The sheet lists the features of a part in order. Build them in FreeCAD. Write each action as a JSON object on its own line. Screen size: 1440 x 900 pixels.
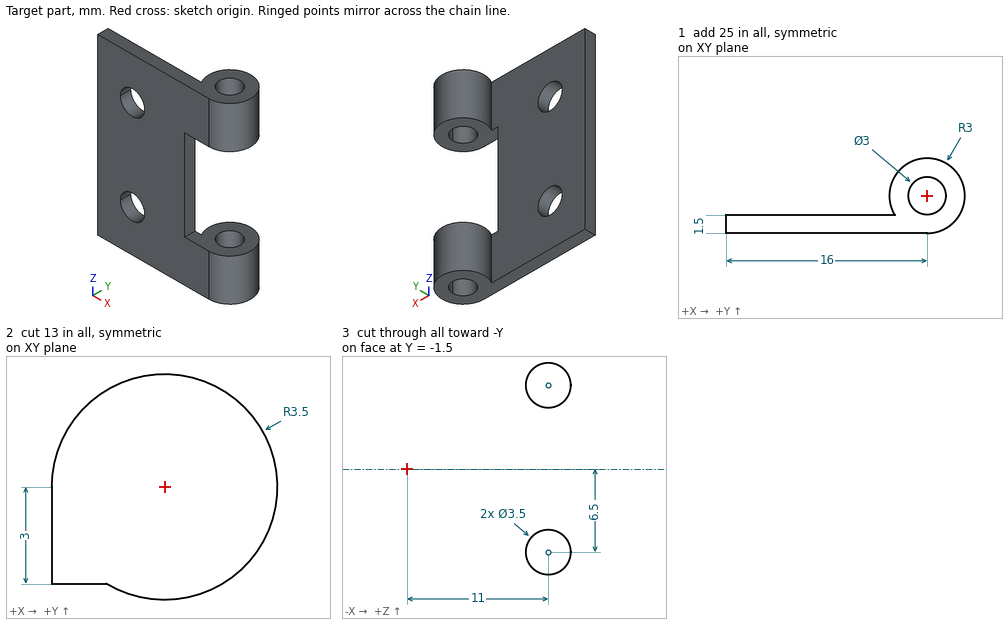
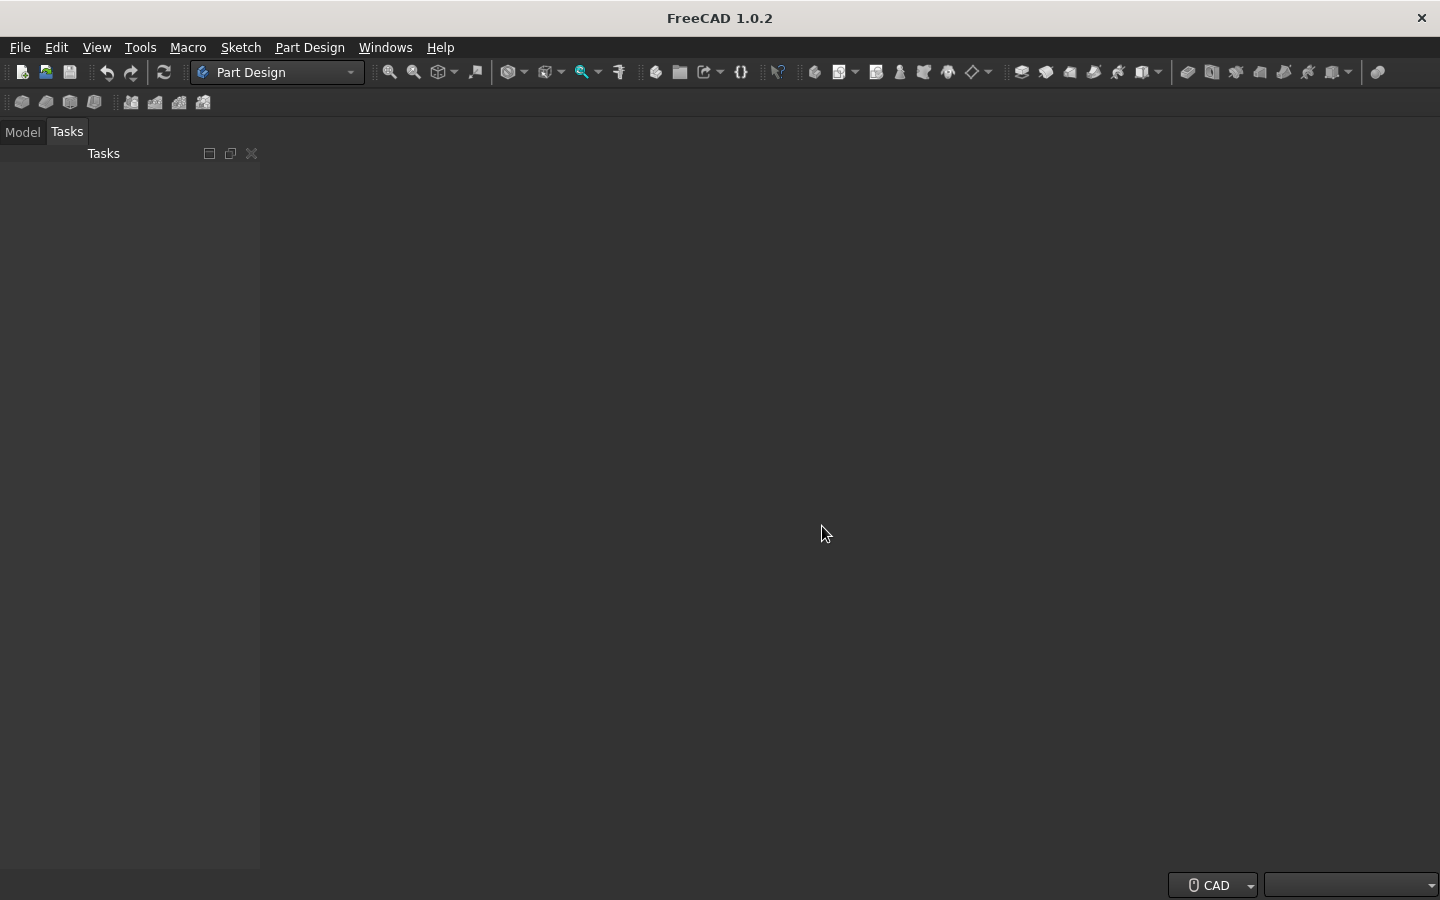
{"action": "left_click", "coordinate": [22, 72]}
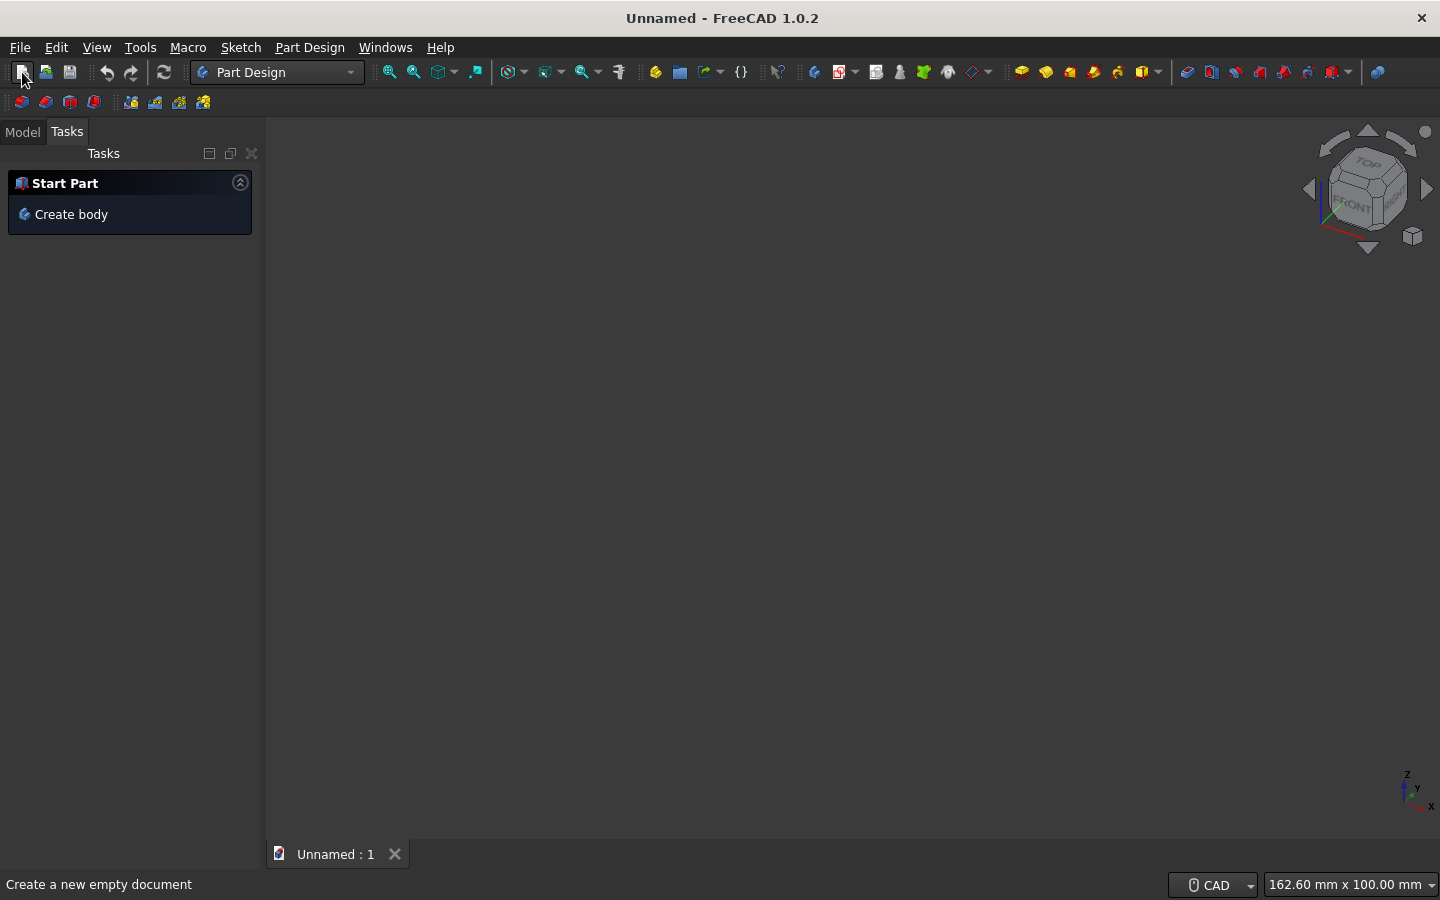
{"action": "left_click", "coordinate": [840, 72]}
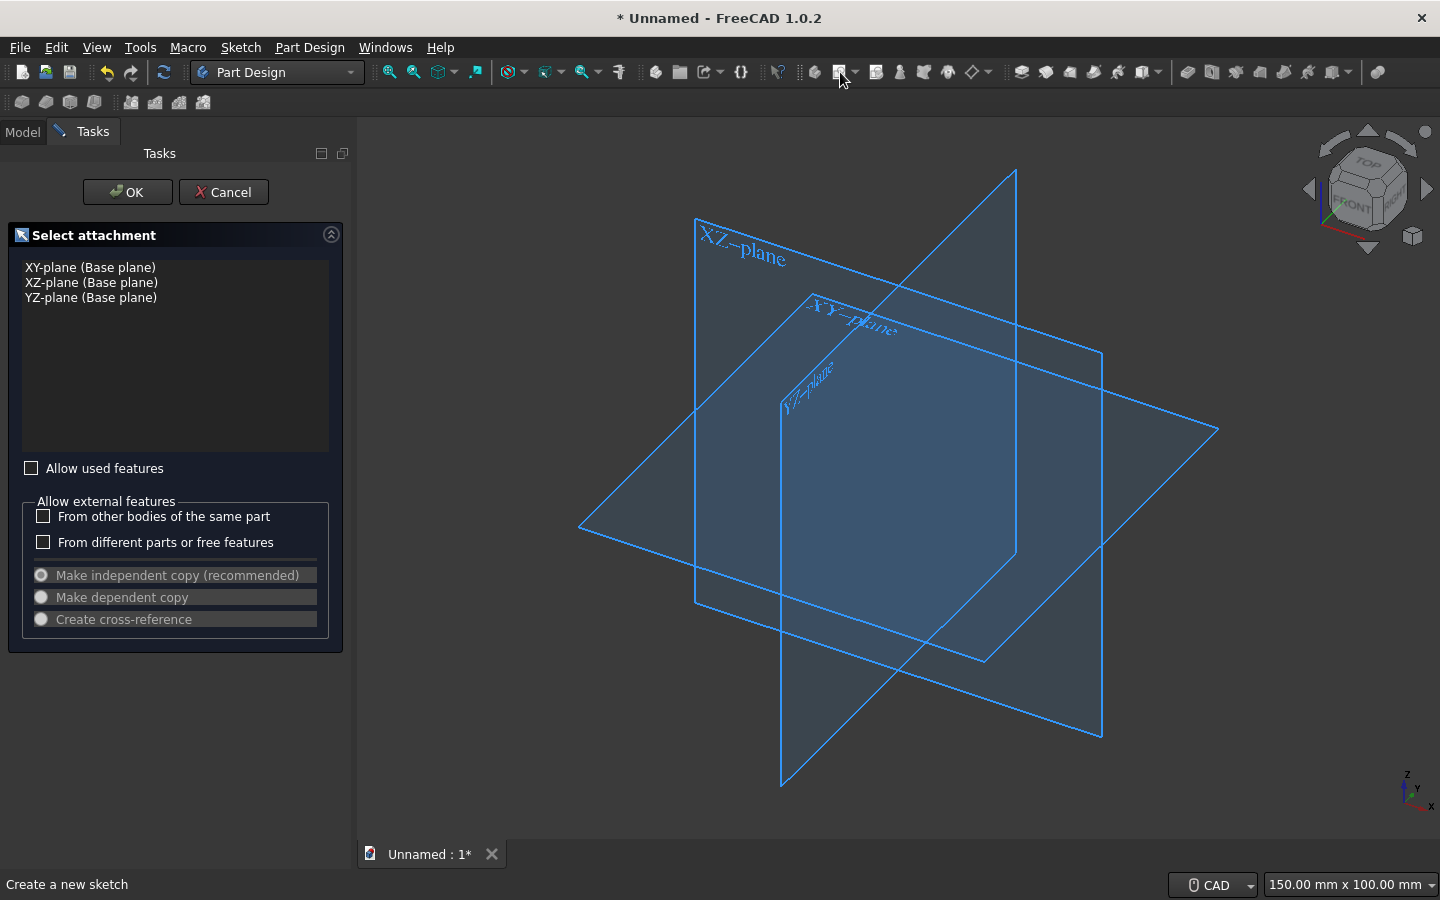
{"action": "left_click", "coordinate": [82, 268]}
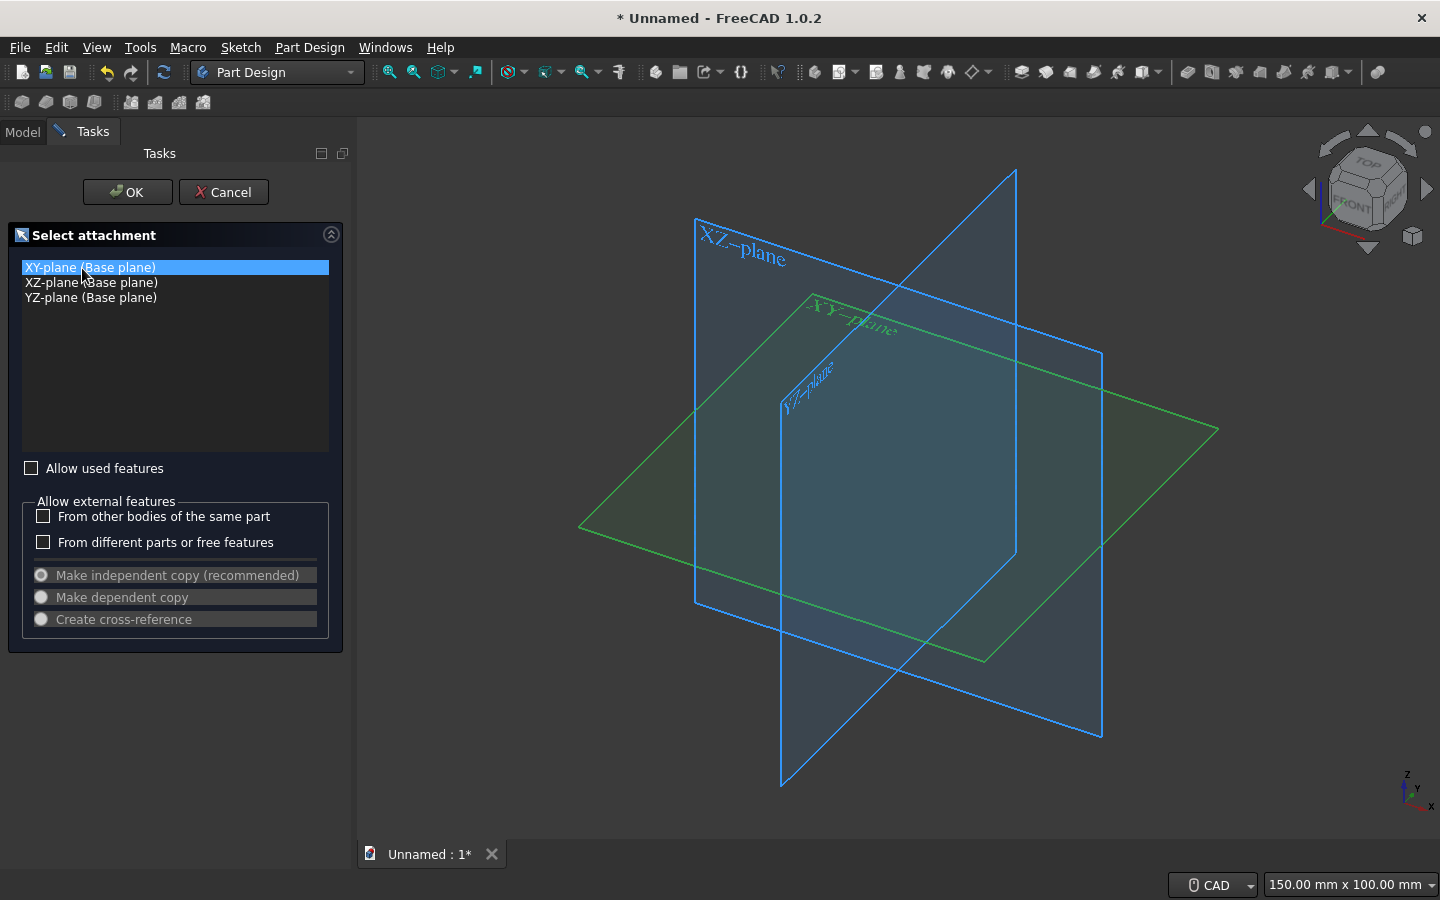
{"action": "left_click", "coordinate": [128, 192]}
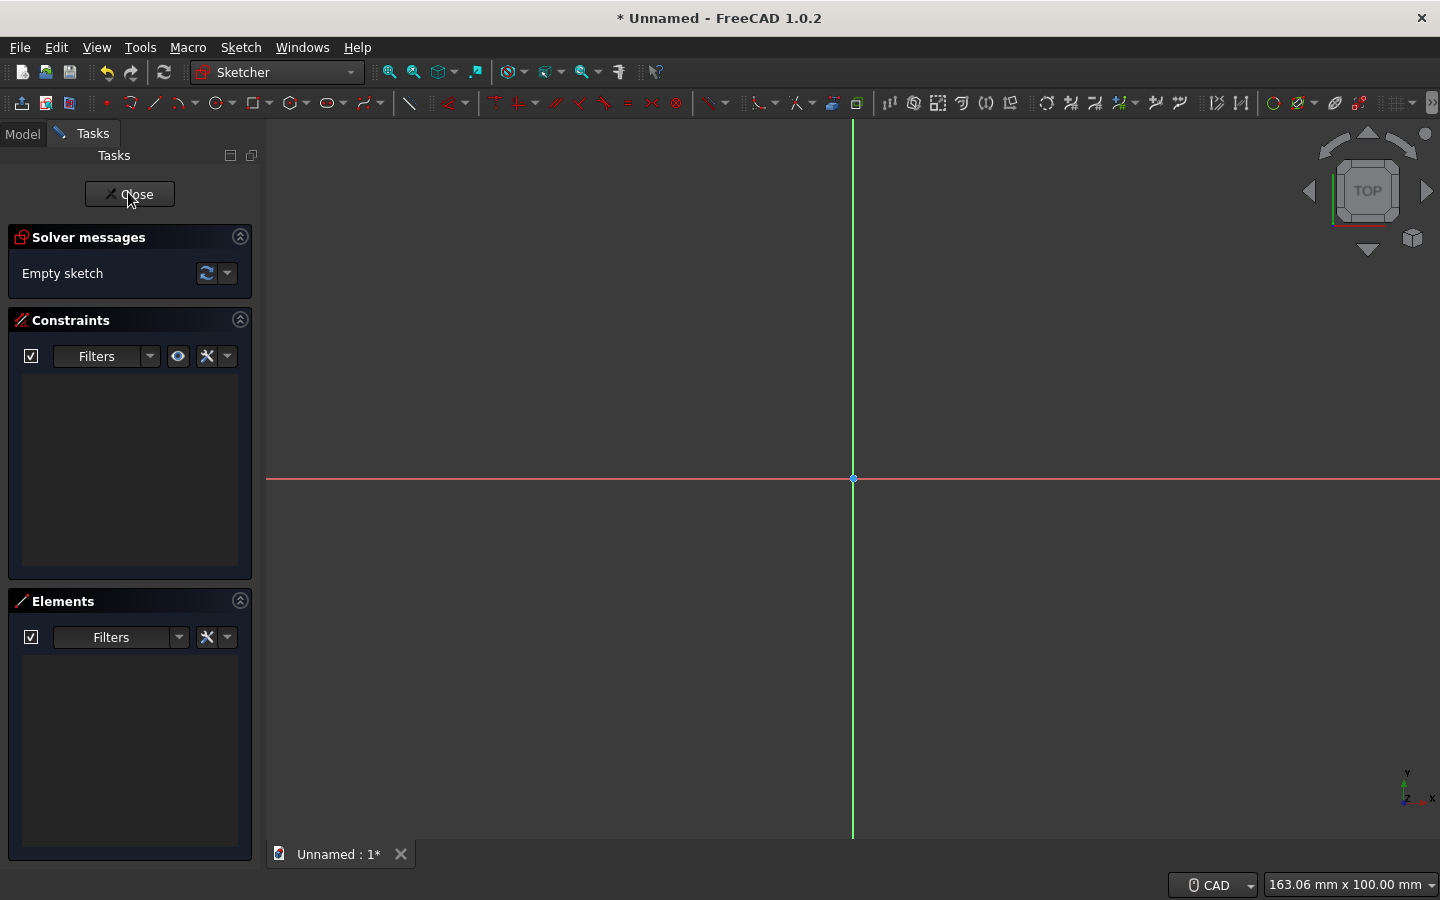
{"action": "scroll", "coordinate": [804, 481], "scroll_direction": "up", "scroll_amount": 9}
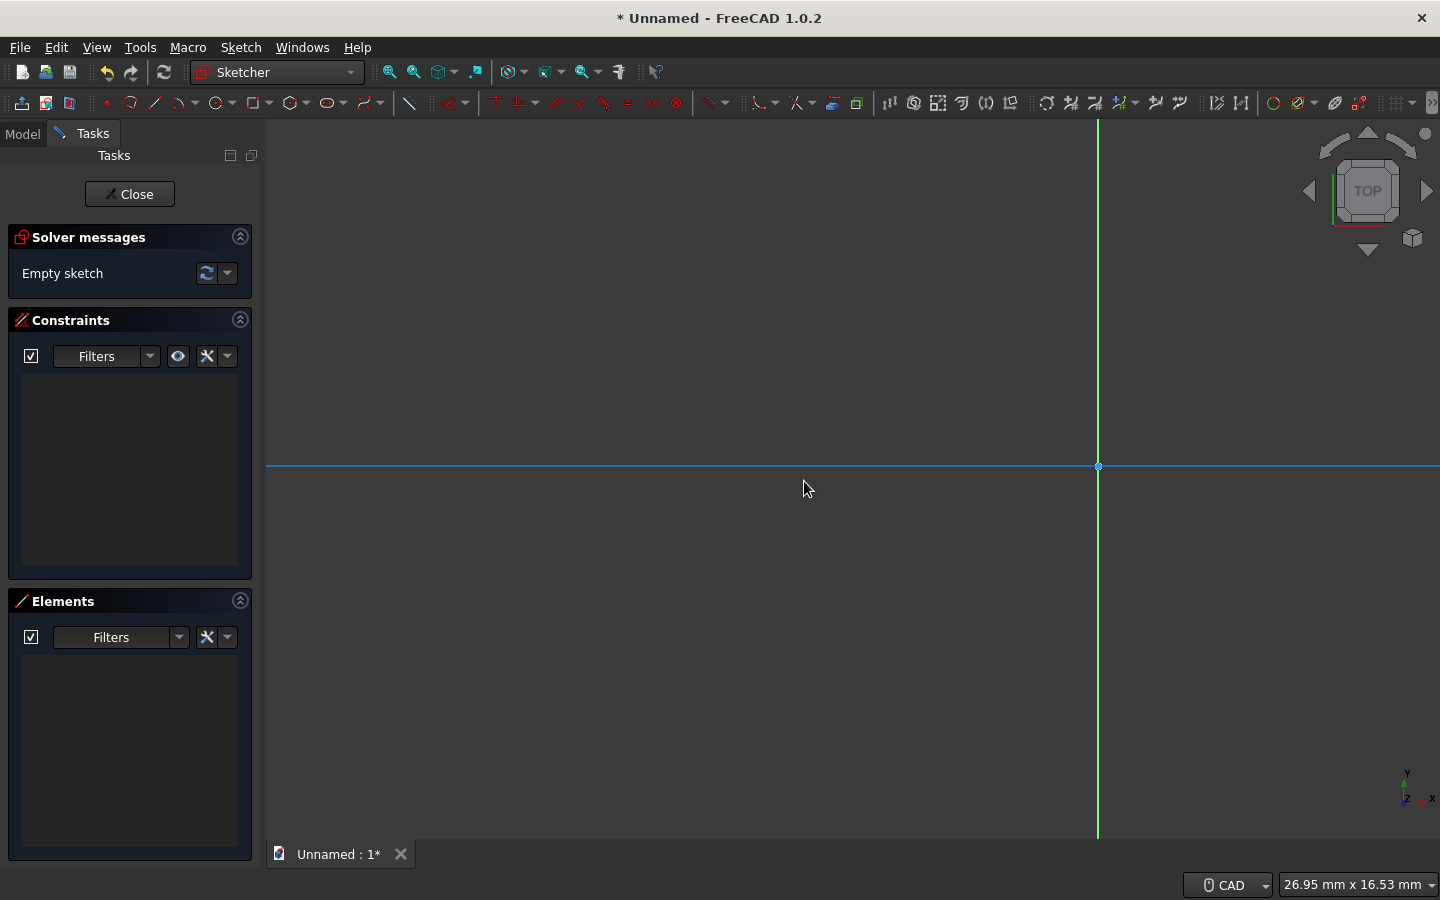
{"action": "left_click", "coordinate": [132, 104]}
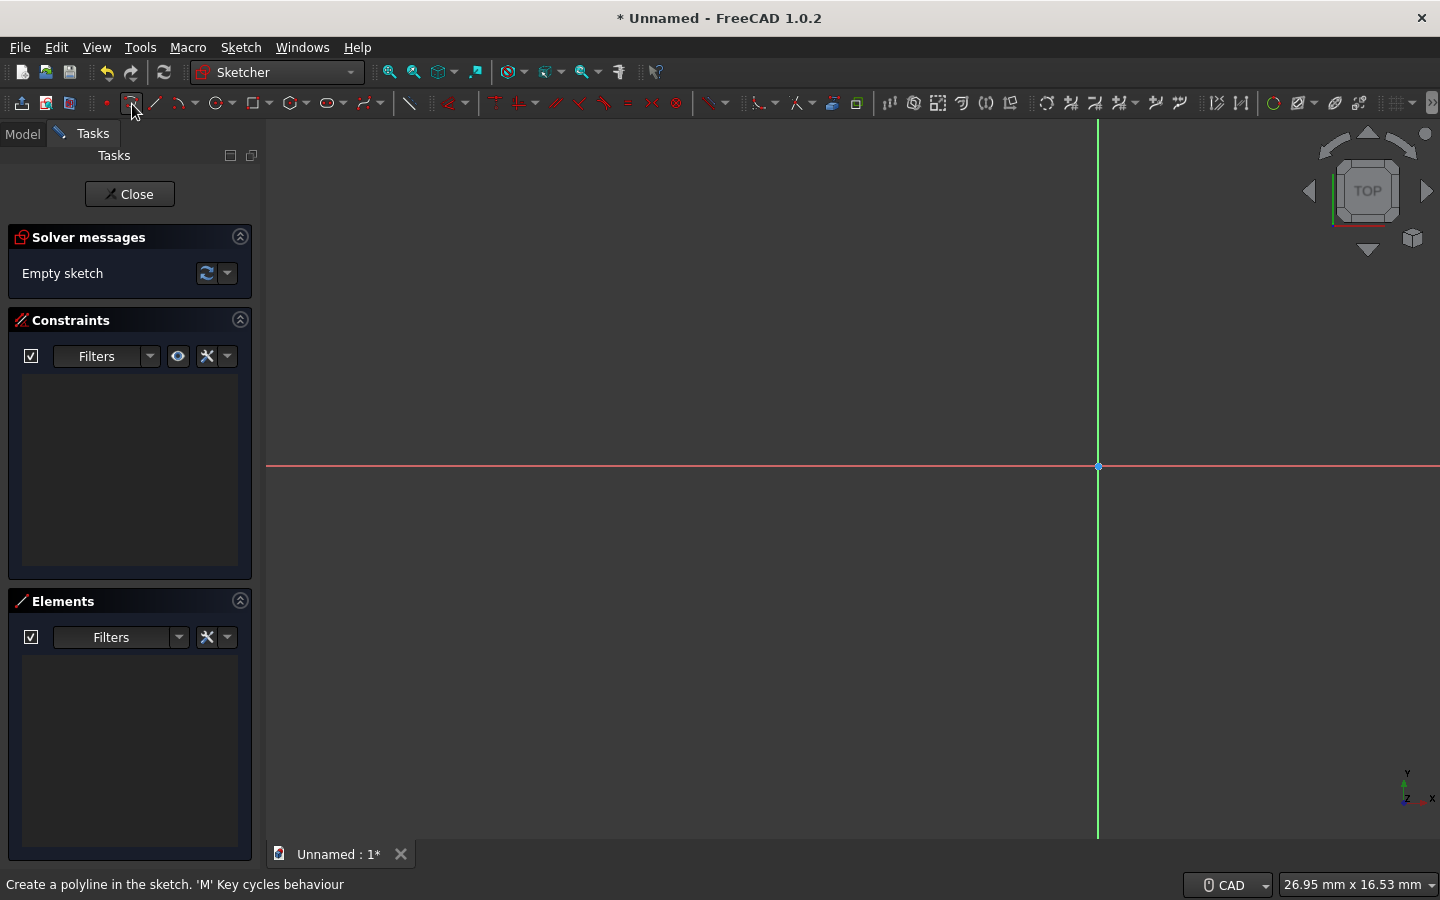
{"action": "left_click", "coordinate": [985, 532]}
{"action": "left_click", "coordinate": [401, 532]}
{"action": "left_click", "coordinate": [401, 597]}
{"action": "left_click", "coordinate": [1098, 597]}
{"action": "right_click", "coordinate": [1098, 597]}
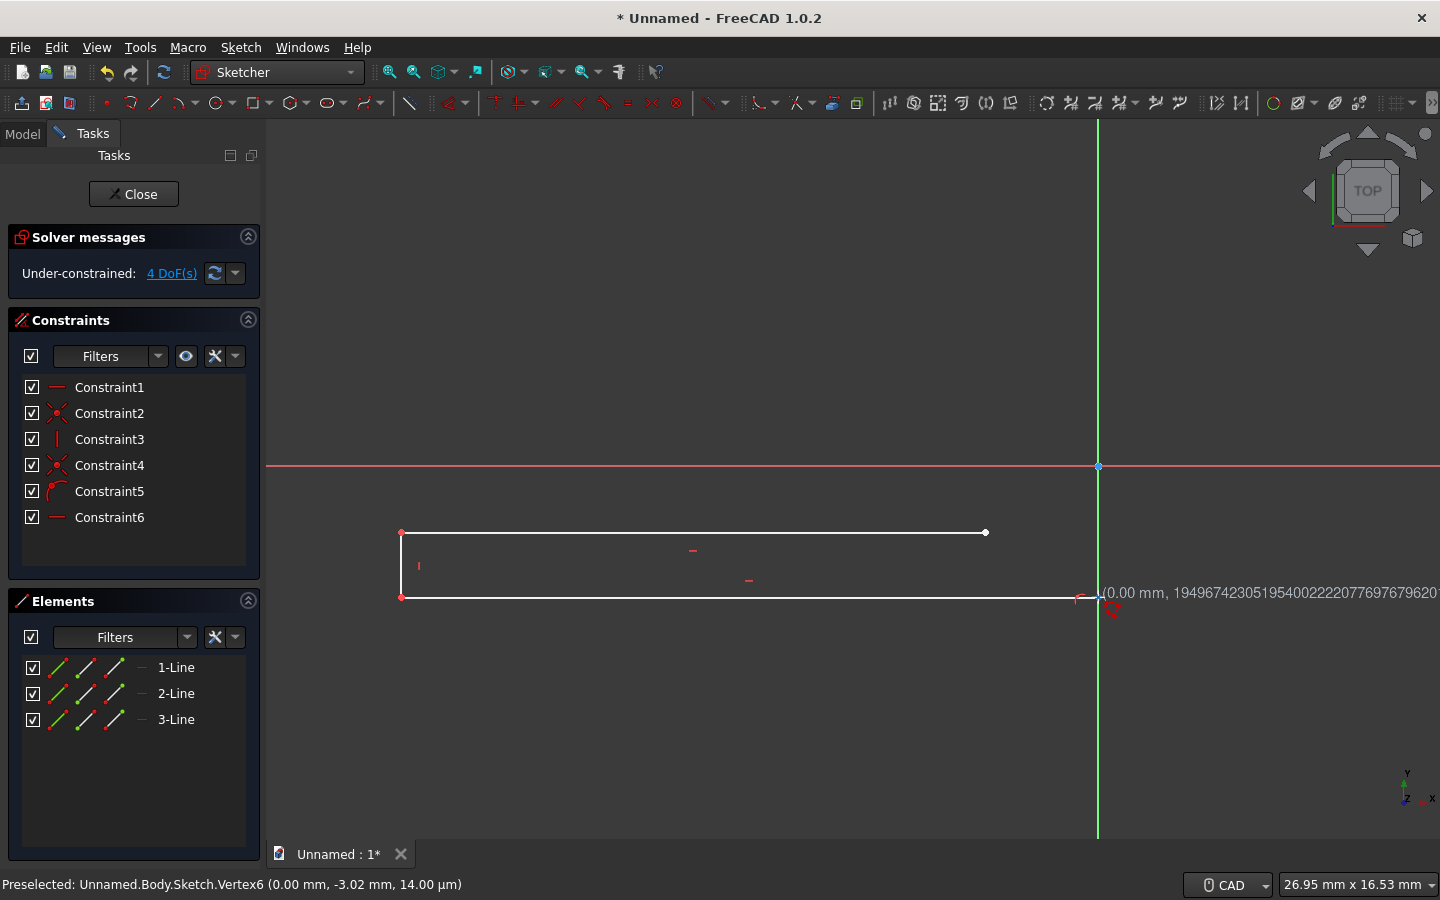
{"action": "left_click", "coordinate": [198, 104]}